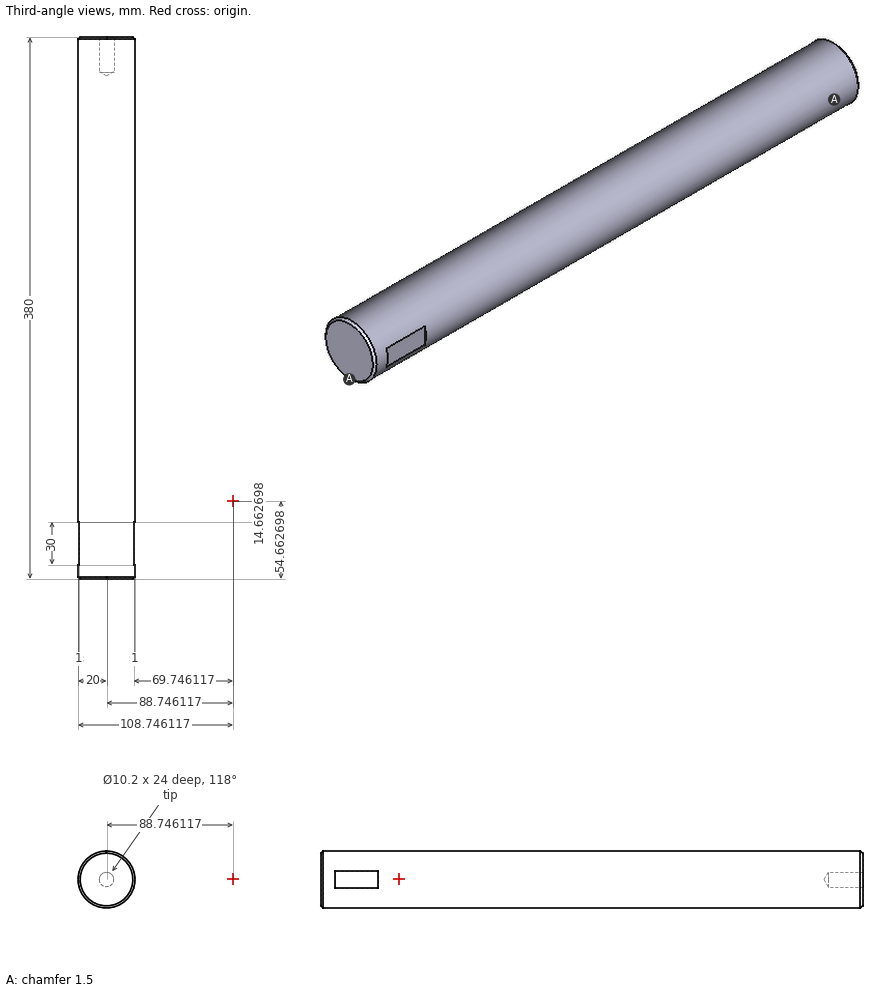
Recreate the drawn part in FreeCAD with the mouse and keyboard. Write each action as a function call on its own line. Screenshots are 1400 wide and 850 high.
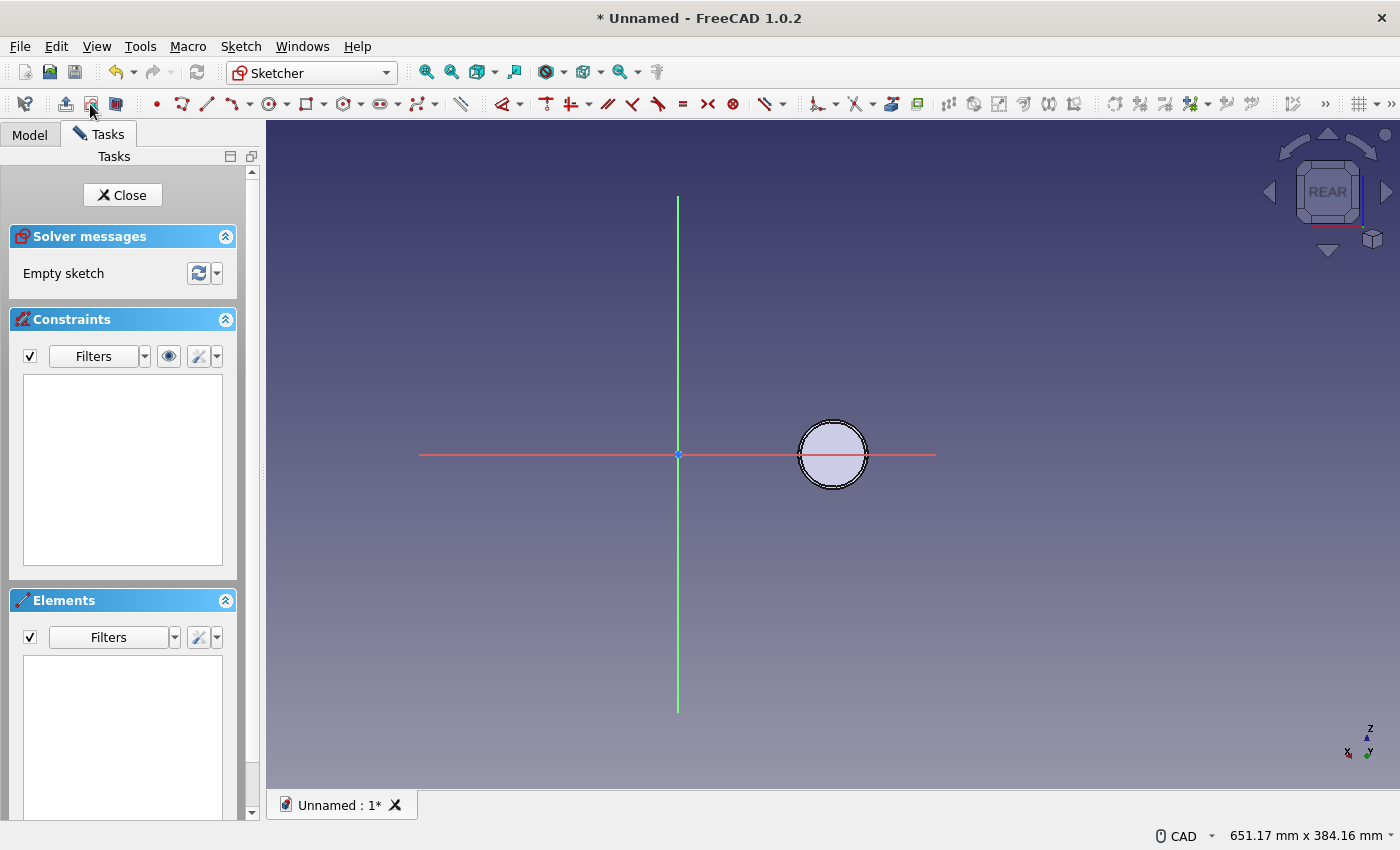
scroll(837, 455, up, 15)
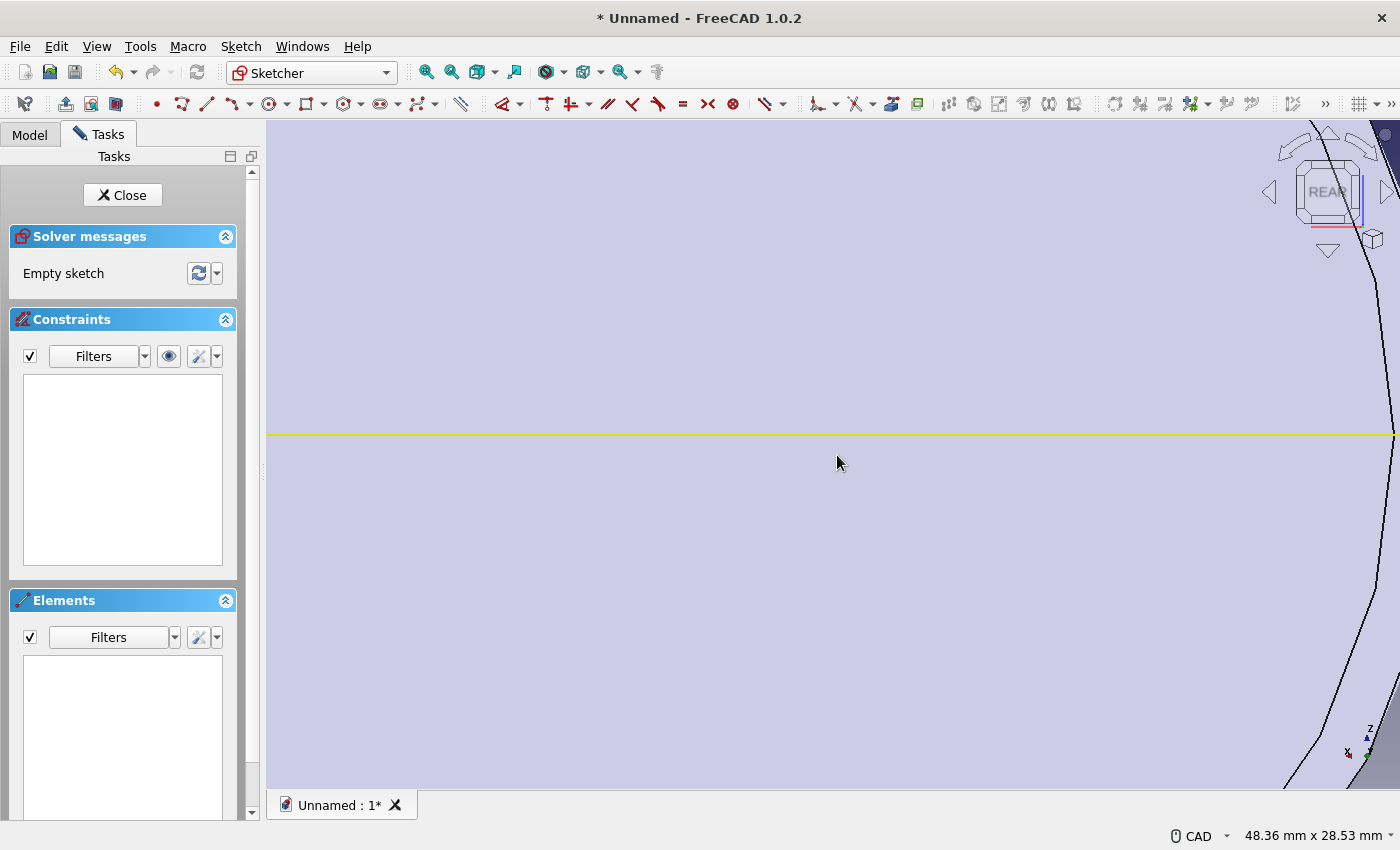
key(g)
key(c)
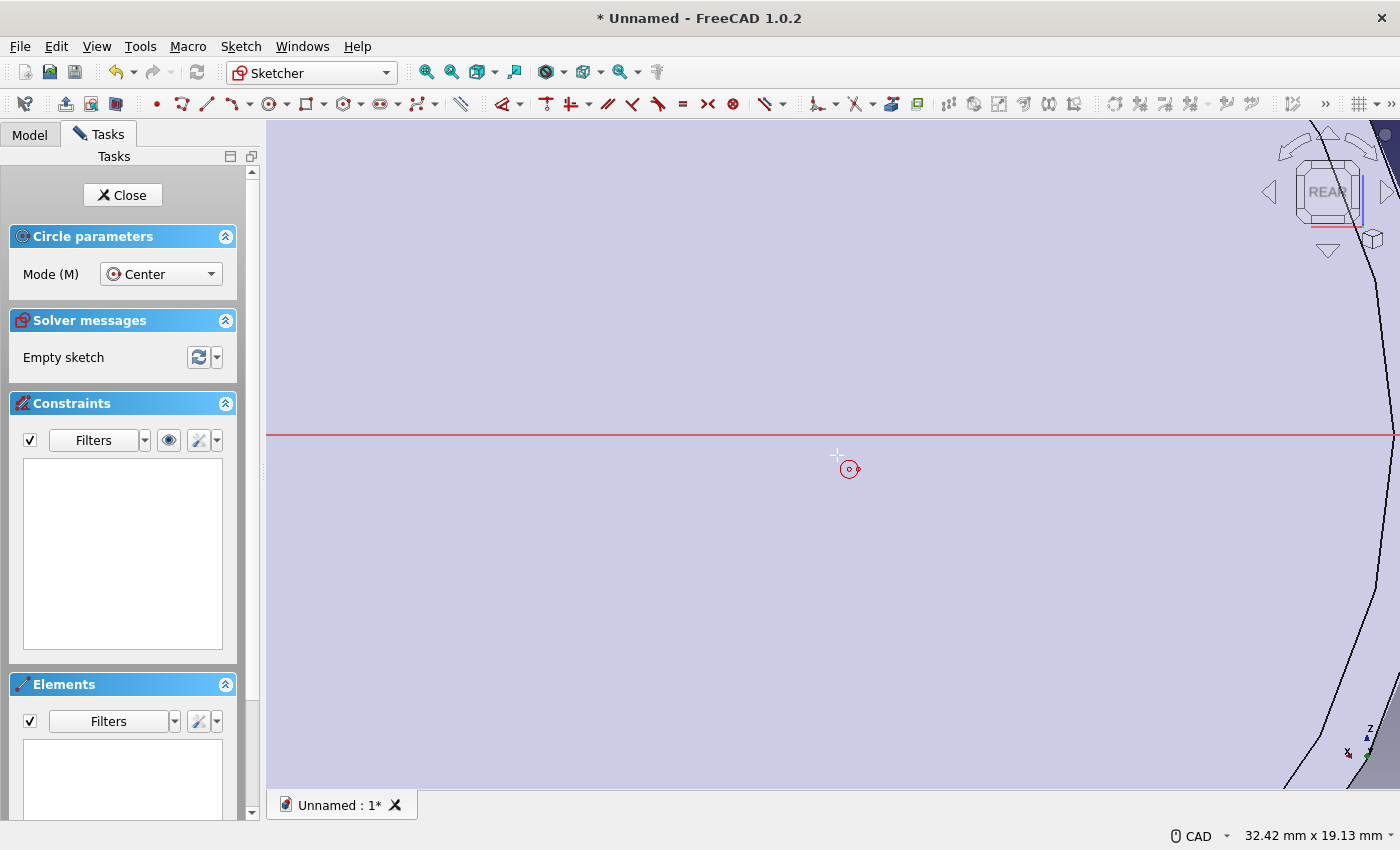
click(747, 435)
move(873, 309)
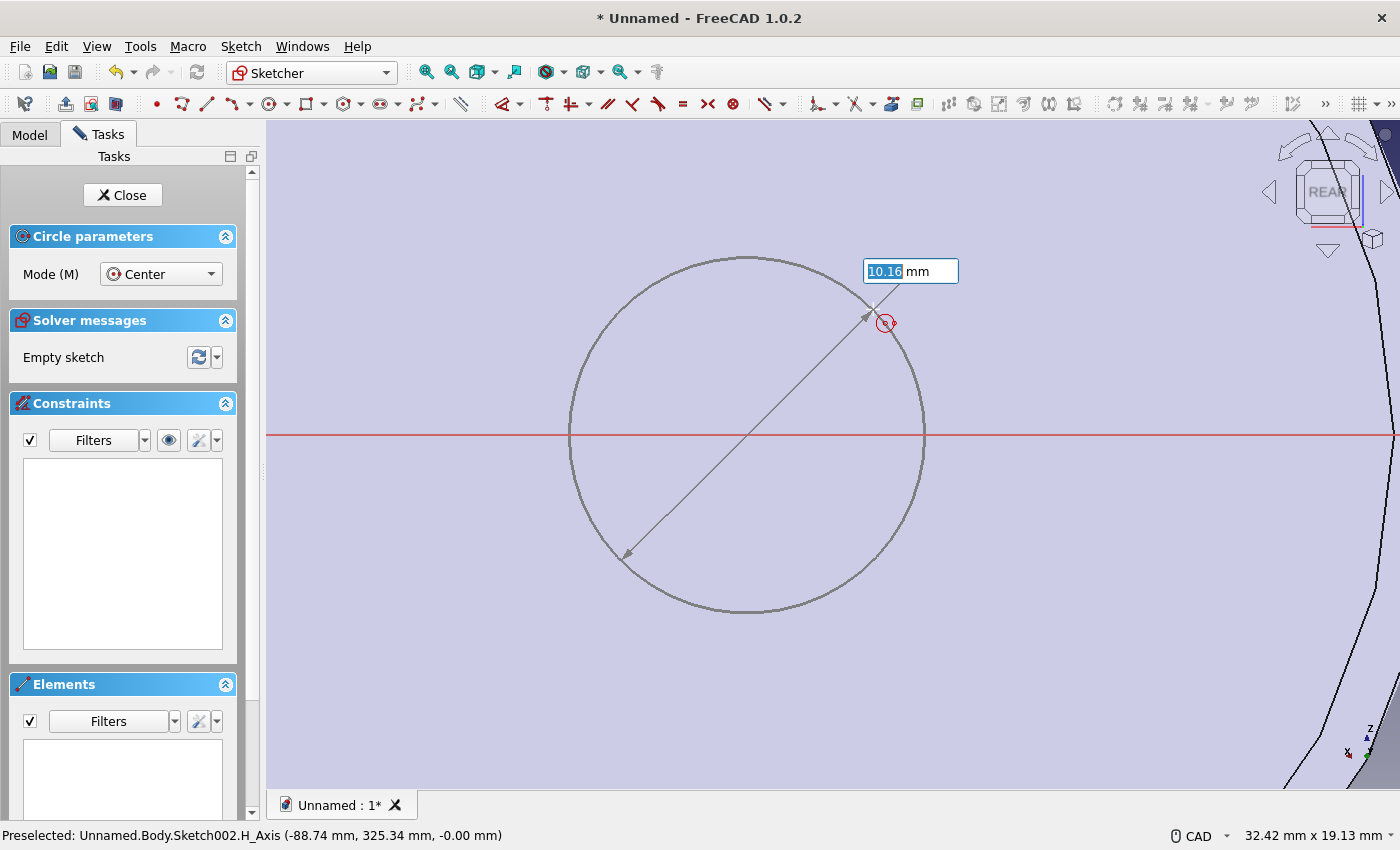
text(10.2)
key(Return)
key(Escape)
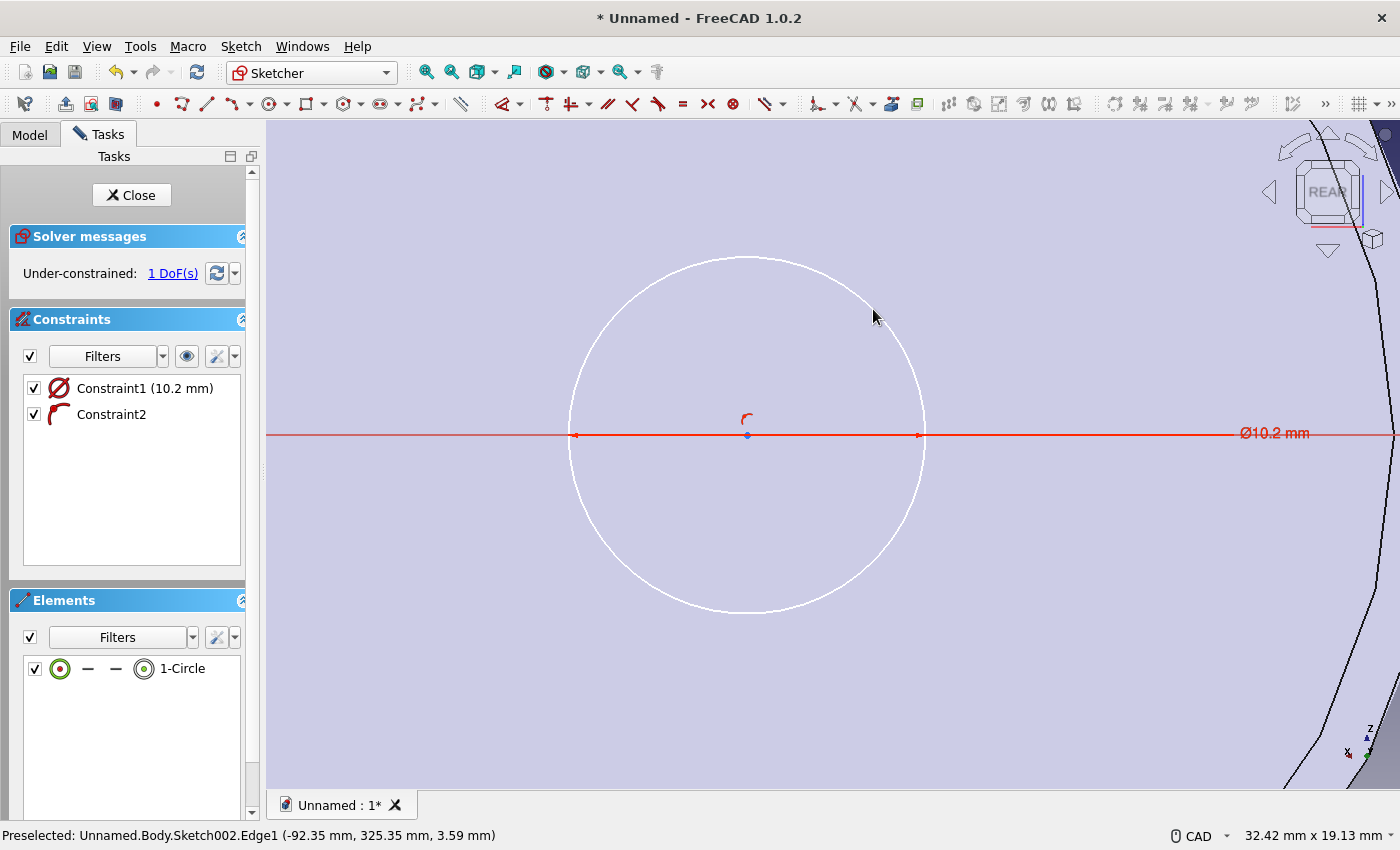
key(d)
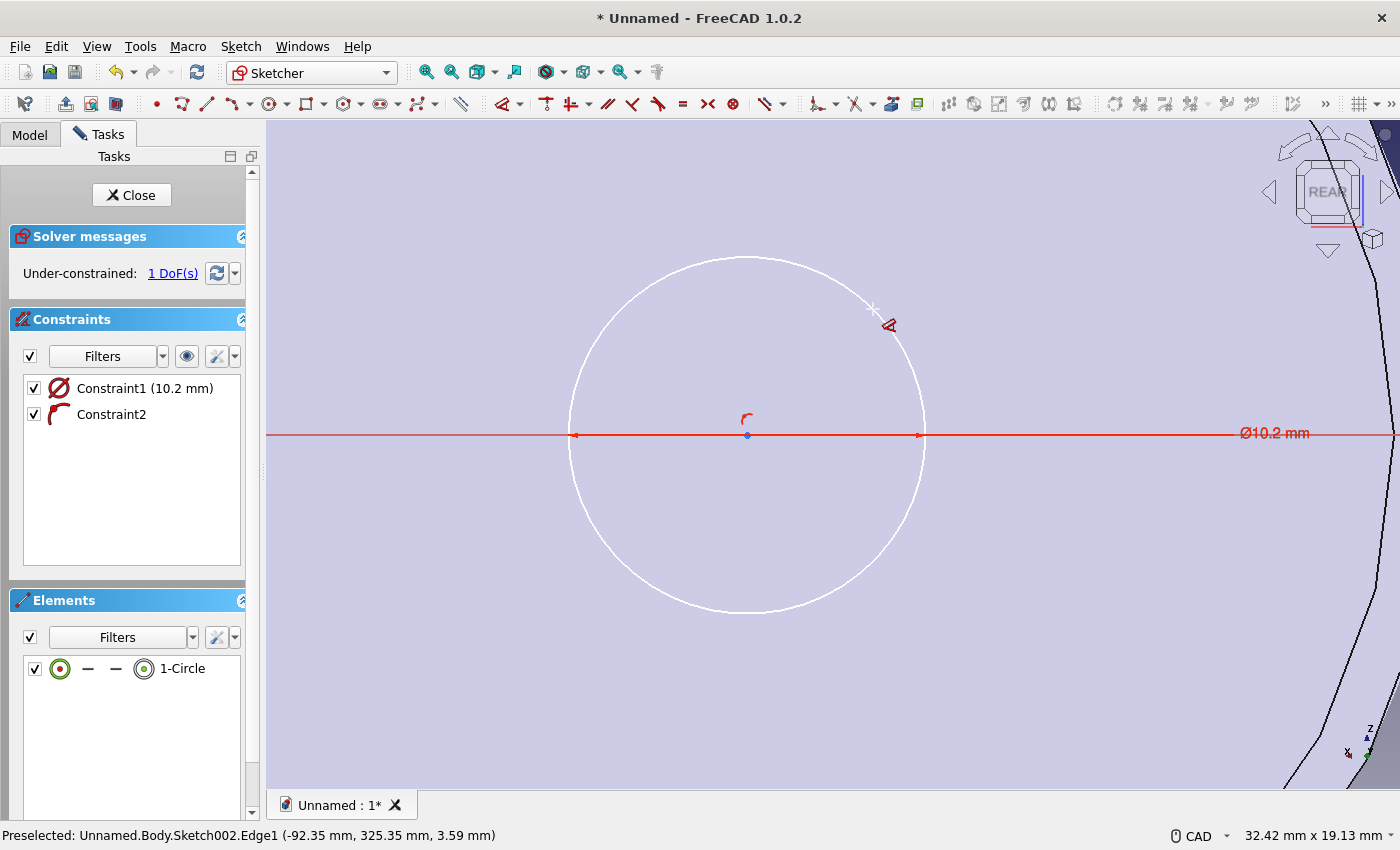
click(747, 435)
click(521, 469)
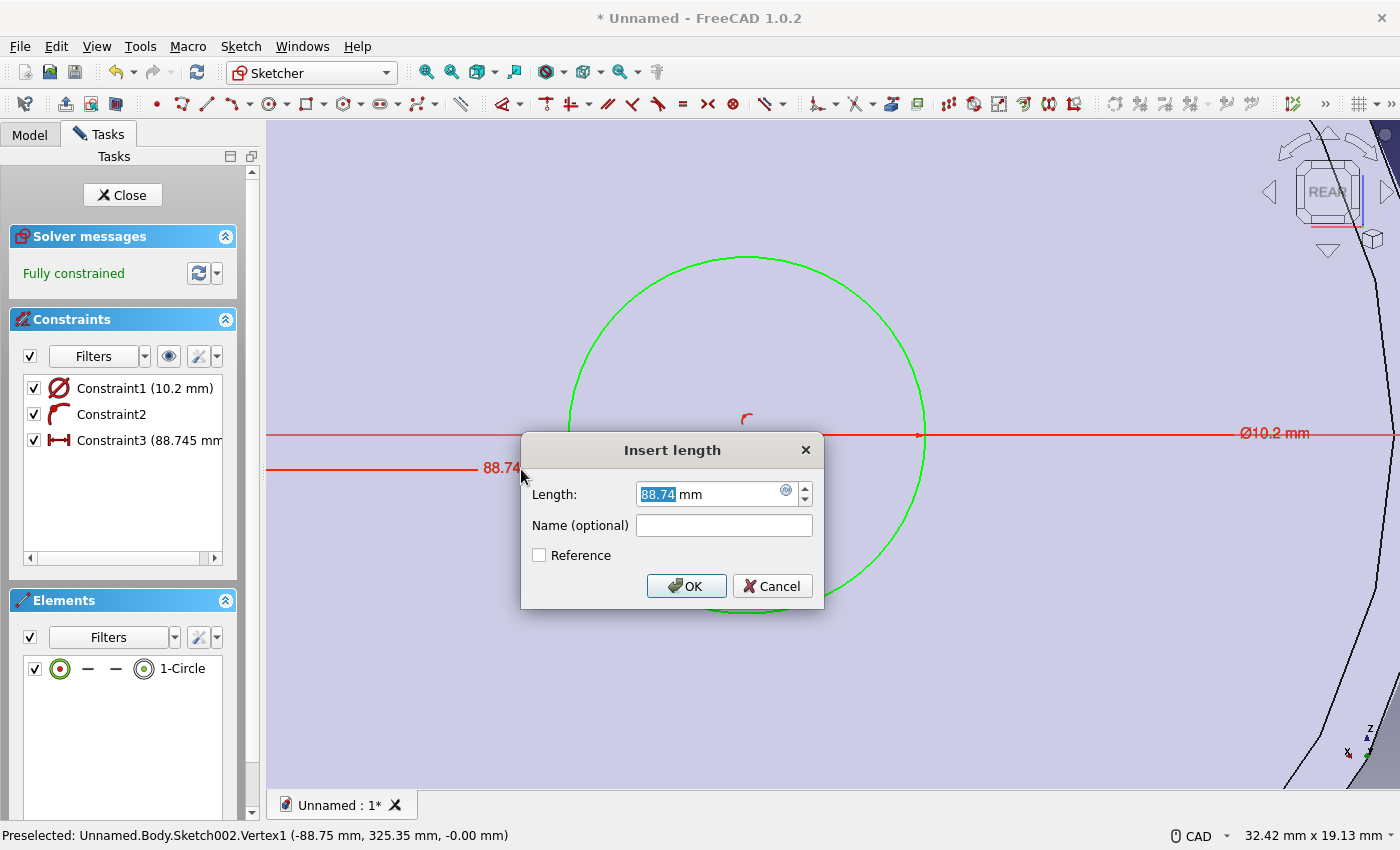
text(88.746117)
key(Return)
key(Escape)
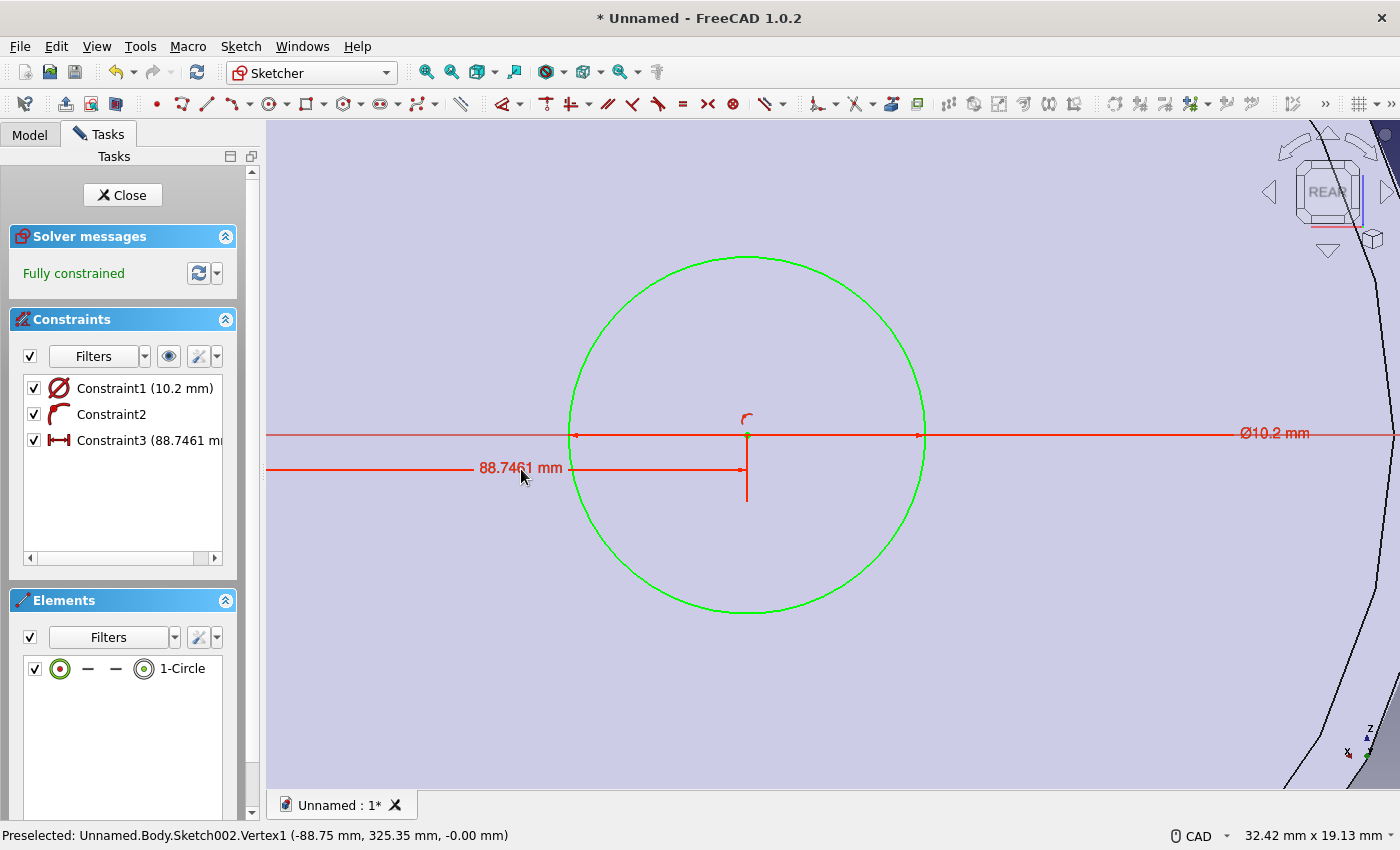
click(123, 195)